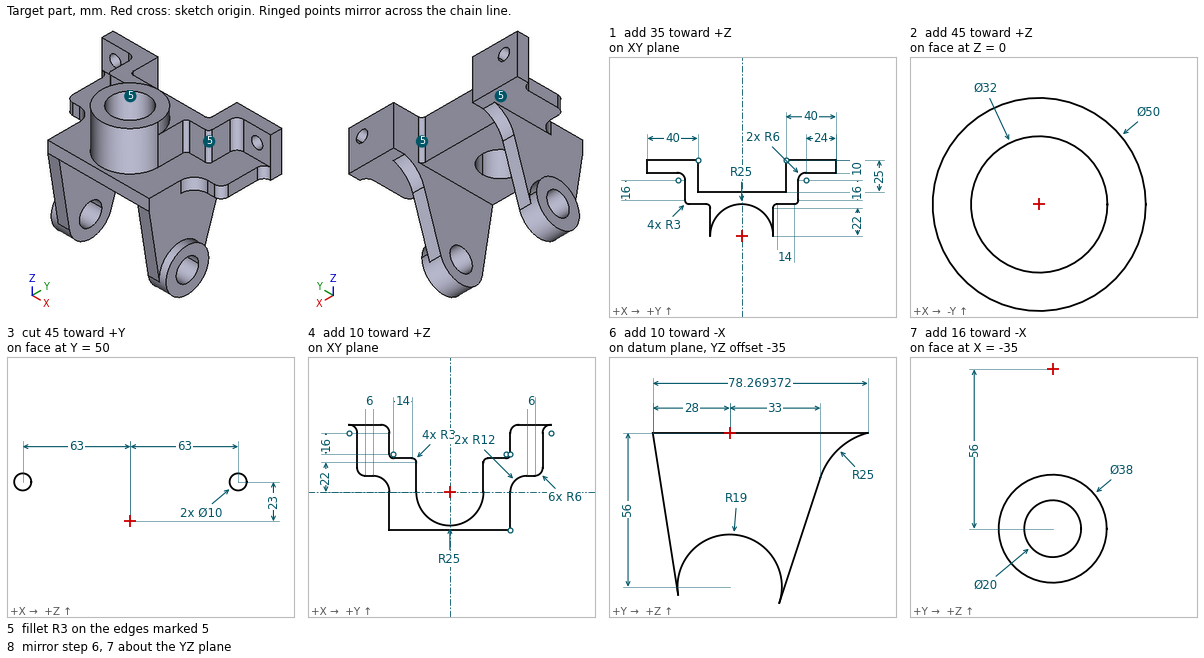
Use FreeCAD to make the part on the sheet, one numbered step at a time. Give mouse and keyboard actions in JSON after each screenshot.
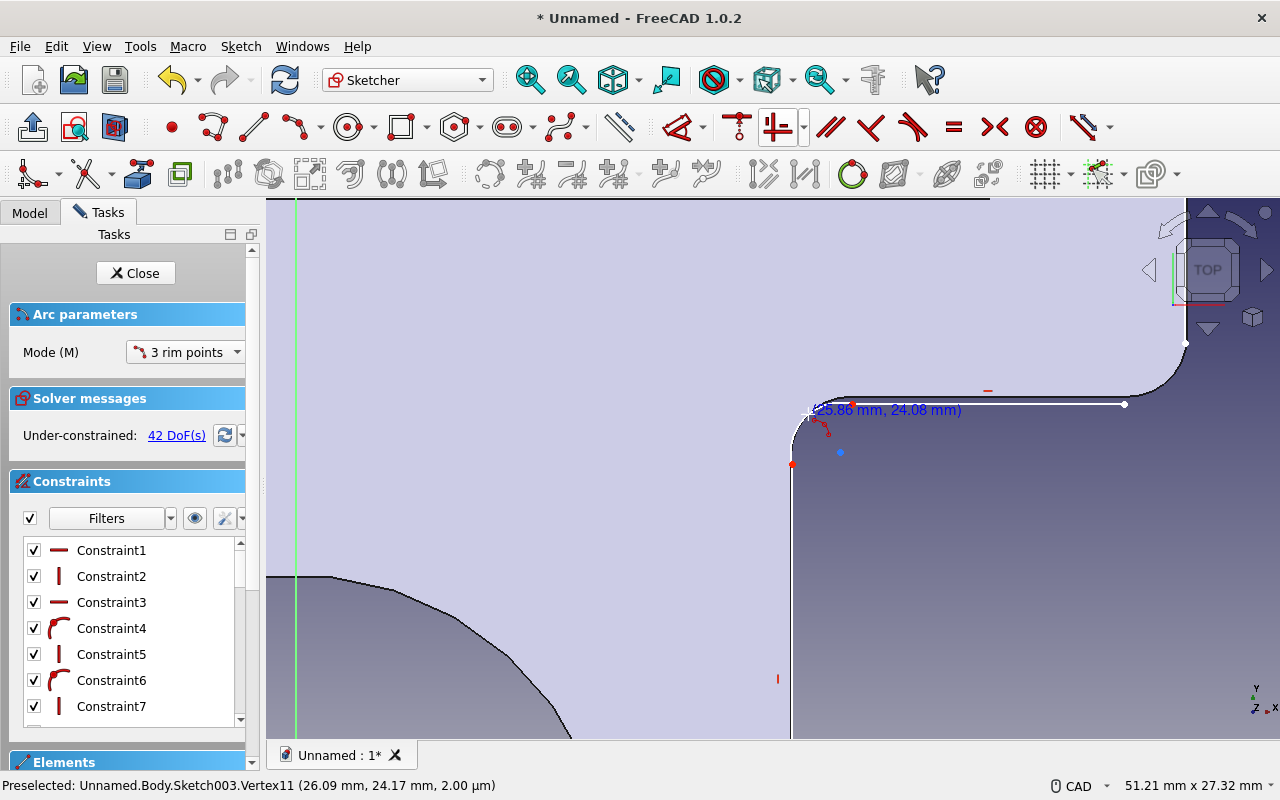
{"action": "scroll", "coordinate": [808, 417], "scroll_direction": "down", "scroll_amount": 8}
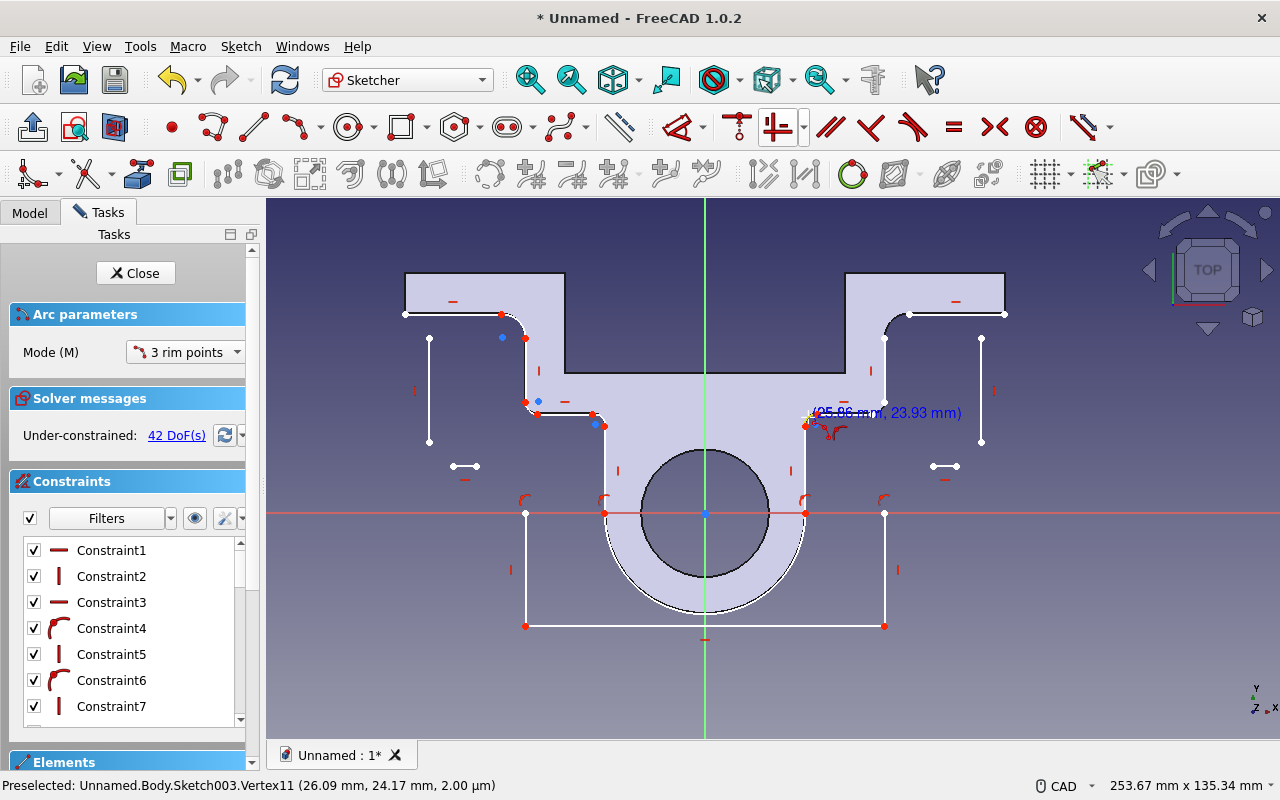
{"action": "left_click", "coordinate": [872, 415]}
{"action": "left_click", "coordinate": [885, 402]}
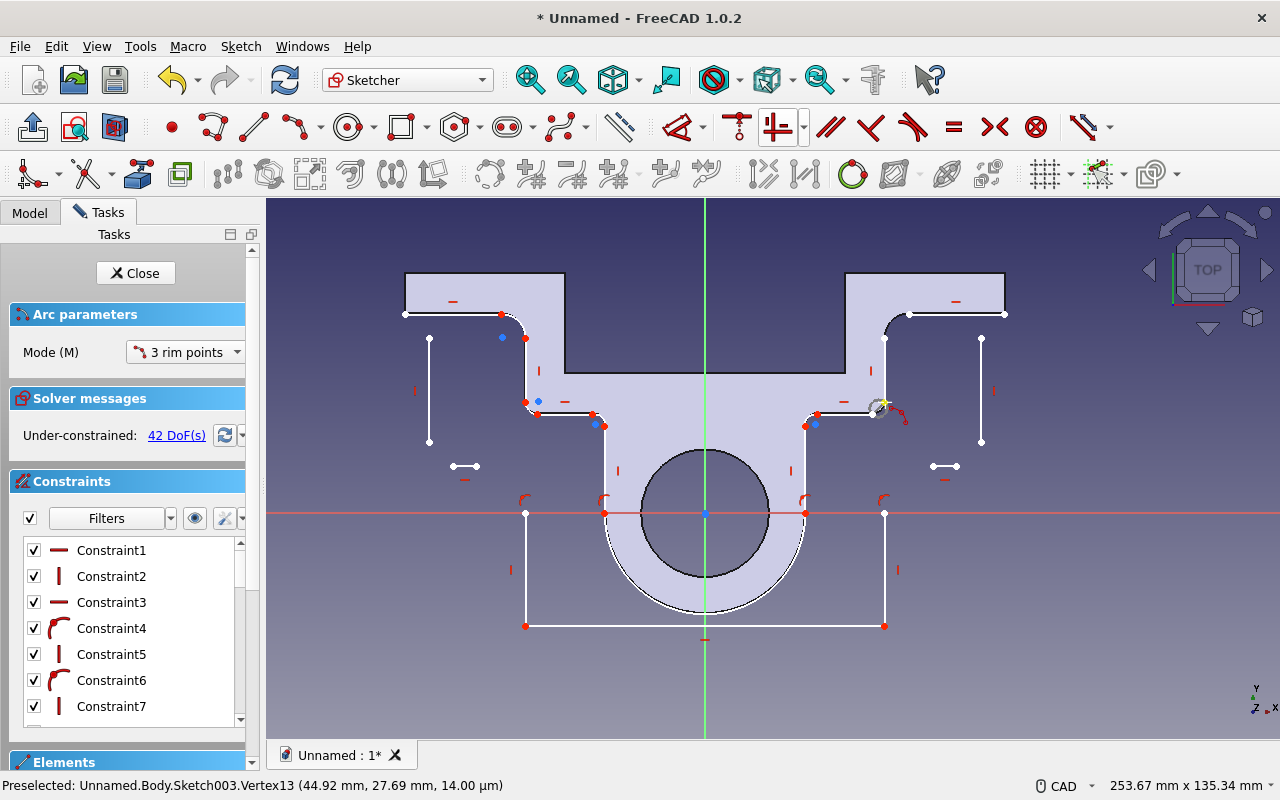
{"action": "scroll", "coordinate": [881, 410], "scroll_direction": "up", "scroll_amount": 8}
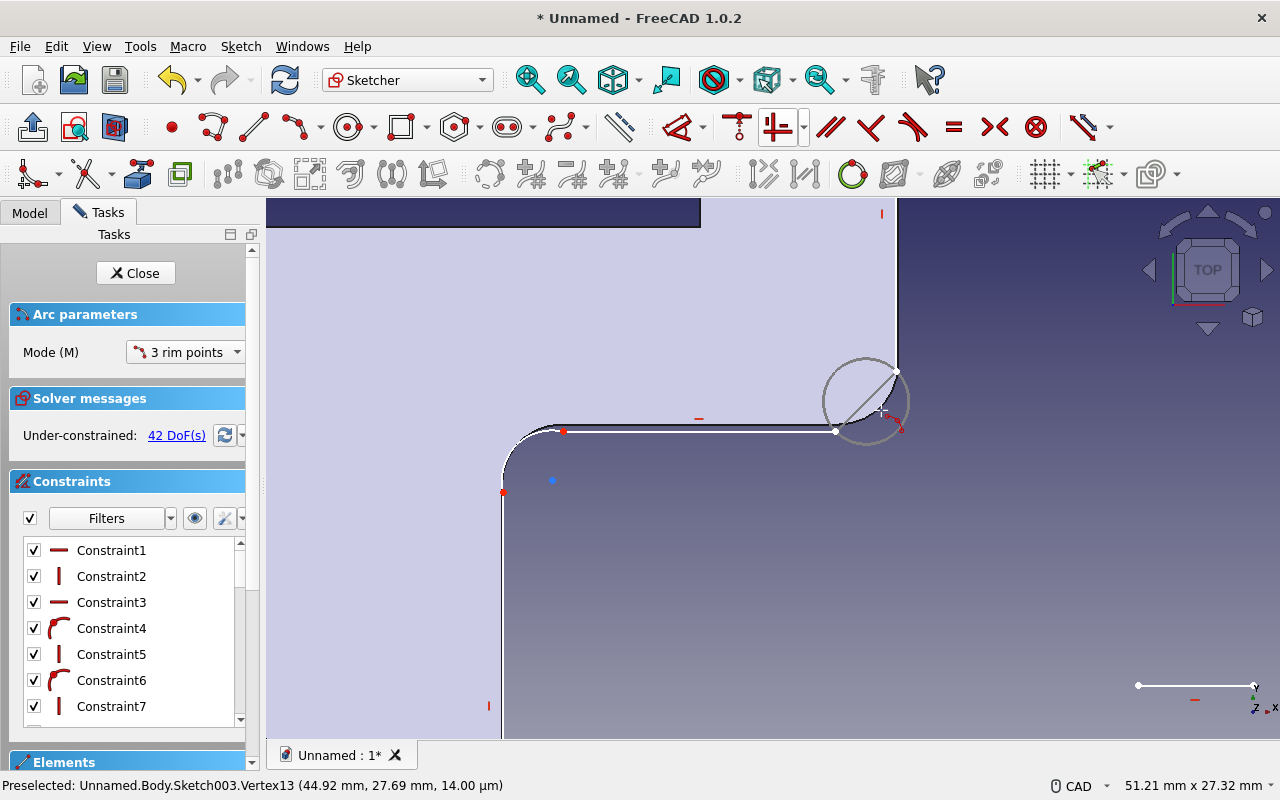
{"action": "left_click", "coordinate": [881, 407]}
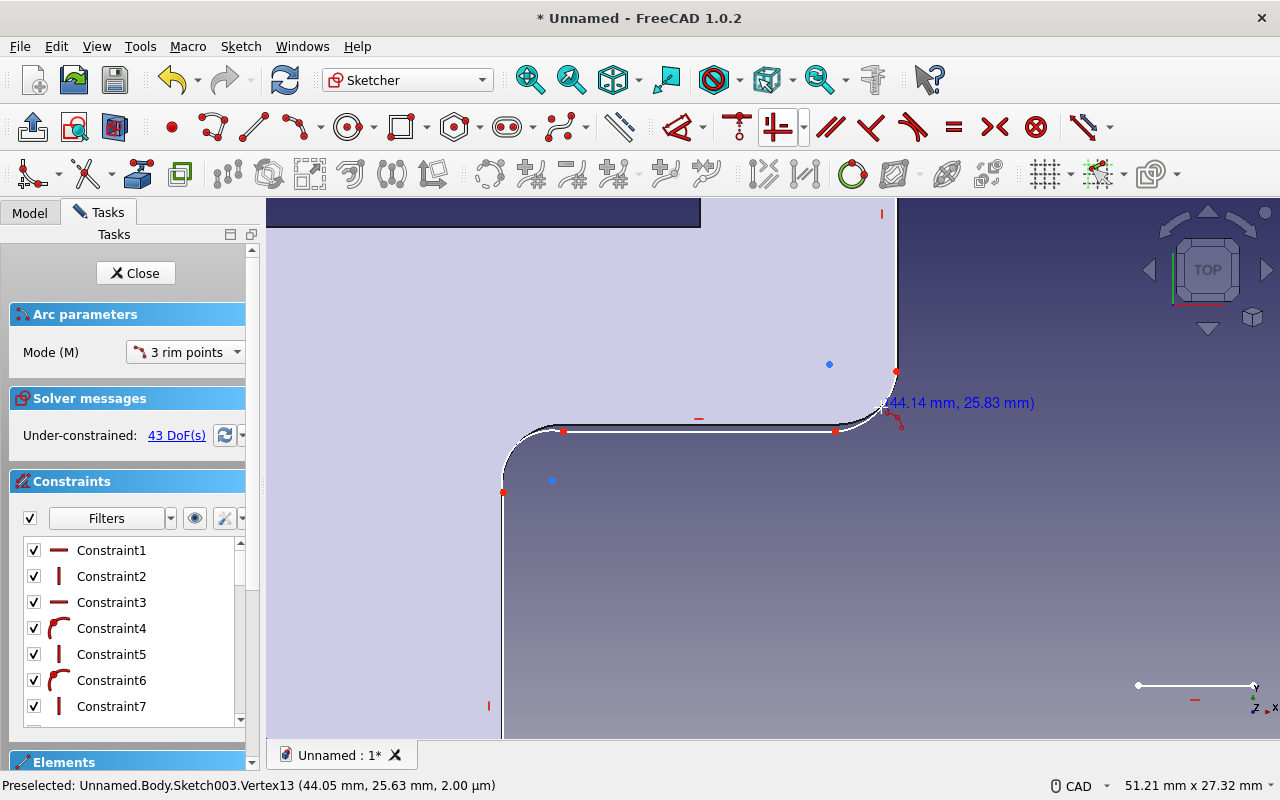
{"action": "scroll", "coordinate": [881, 410], "scroll_direction": "down", "scroll_amount": 8}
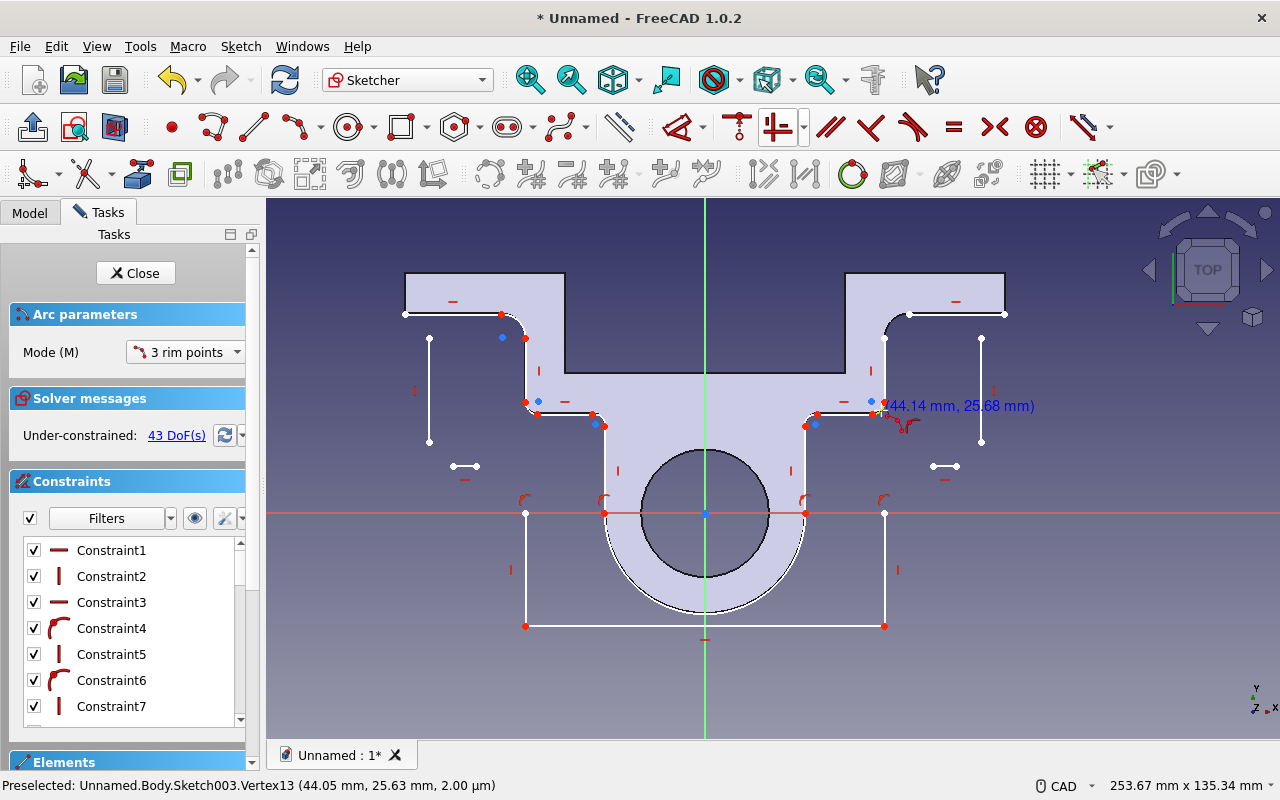
{"action": "left_click", "coordinate": [885, 339]}
{"action": "left_click", "coordinate": [909, 315]}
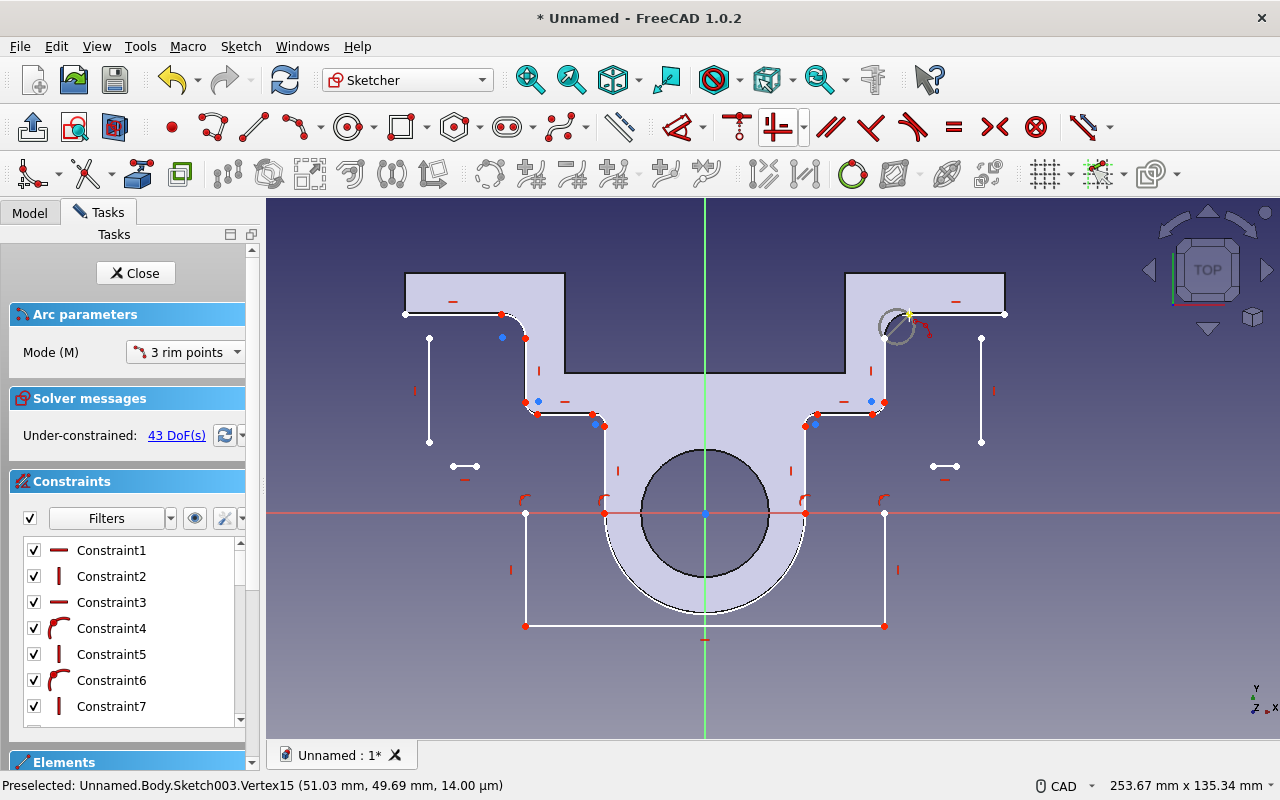
{"action": "scroll", "coordinate": [892, 320], "scroll_direction": "up", "scroll_amount": 5}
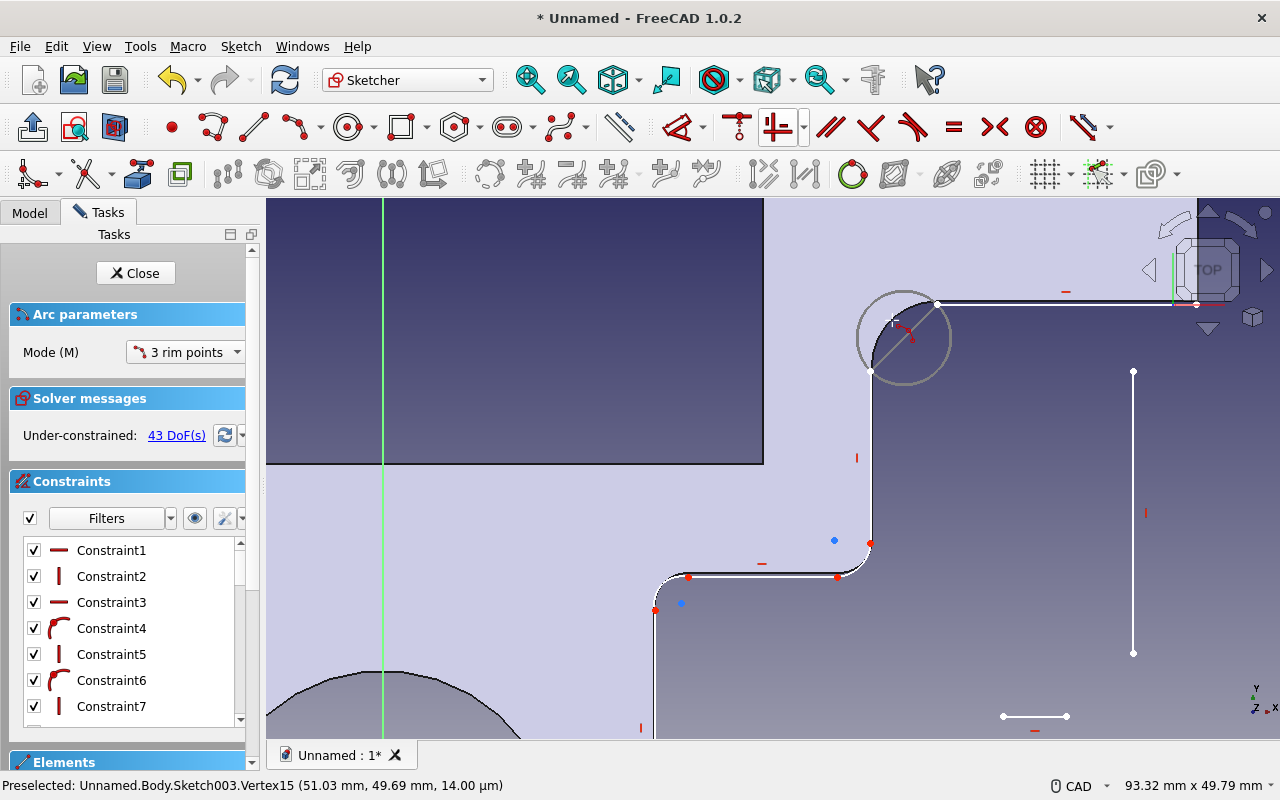
{"action": "left_click", "coordinate": [891, 321]}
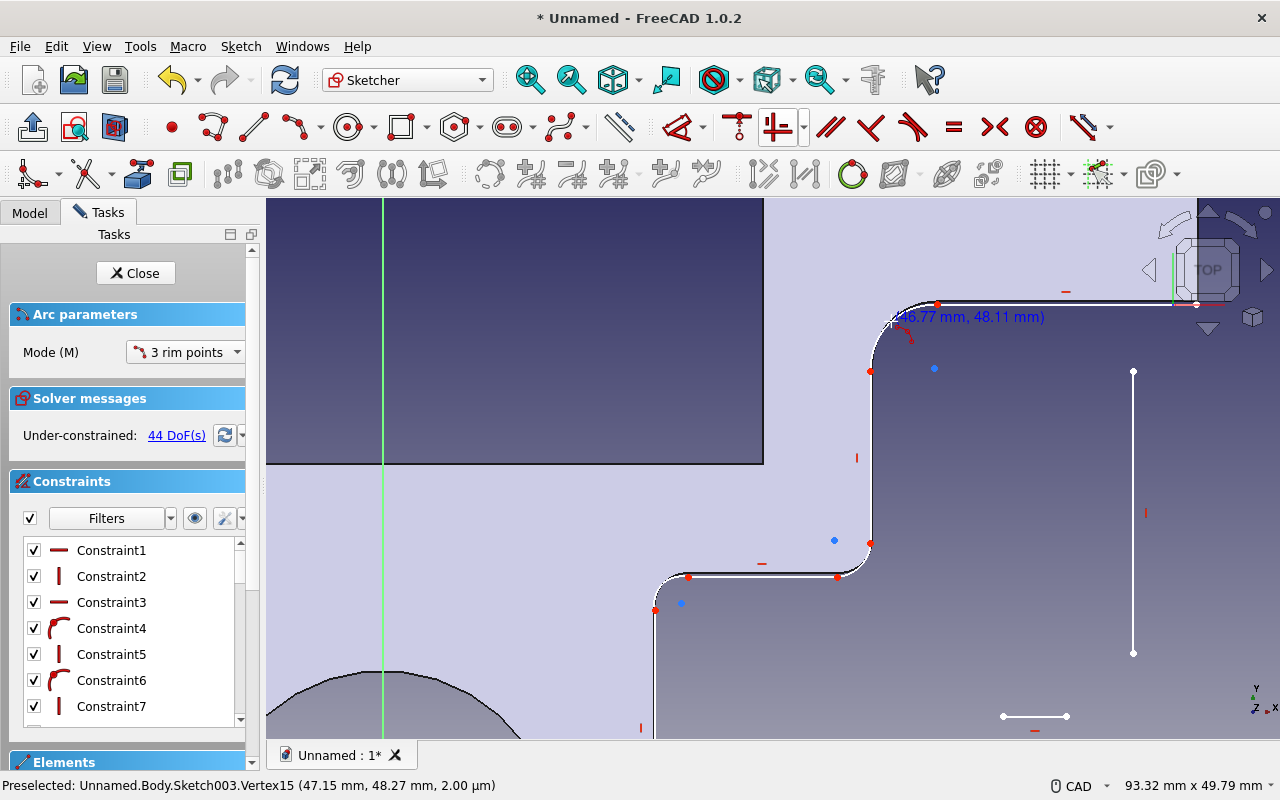
{"action": "scroll", "coordinate": [892, 319], "scroll_direction": "down", "scroll_amount": 5}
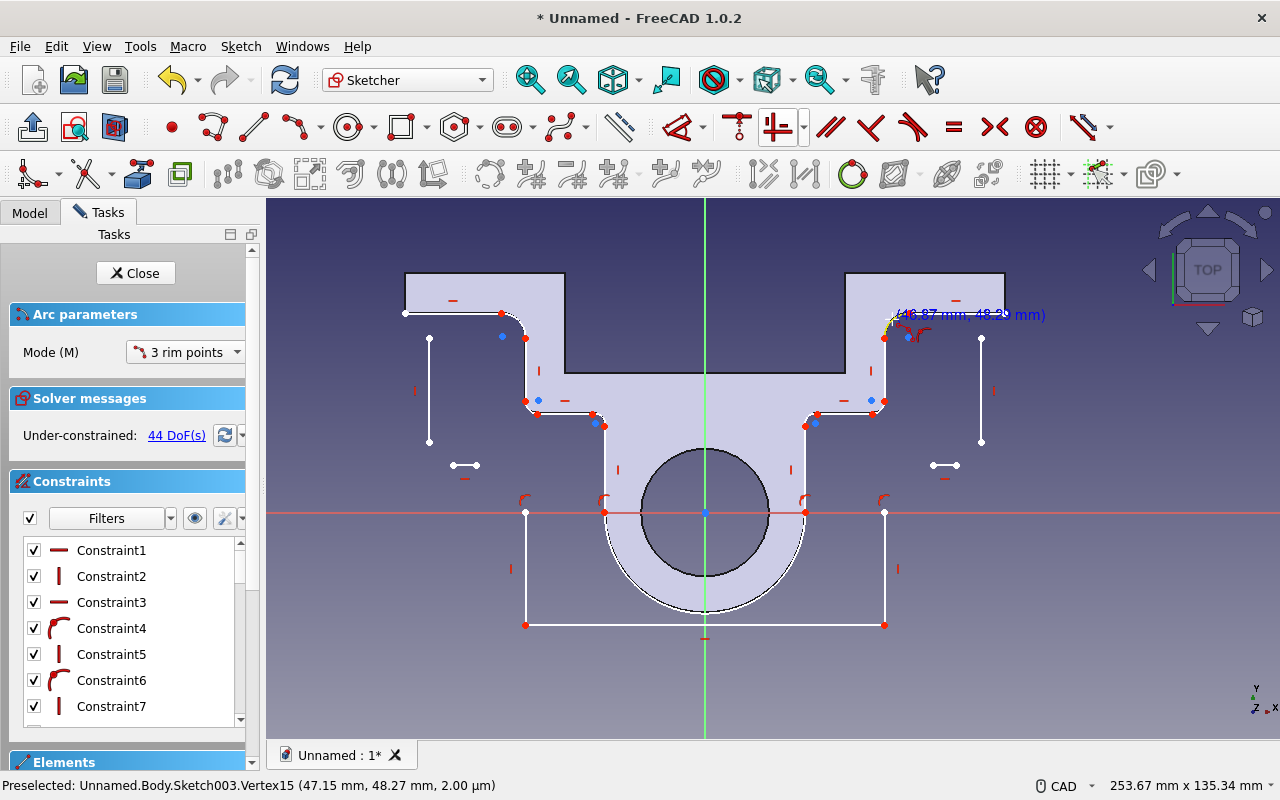
{"action": "left_click", "coordinate": [1004, 314]}
{"action": "left_click", "coordinate": [981, 338]}